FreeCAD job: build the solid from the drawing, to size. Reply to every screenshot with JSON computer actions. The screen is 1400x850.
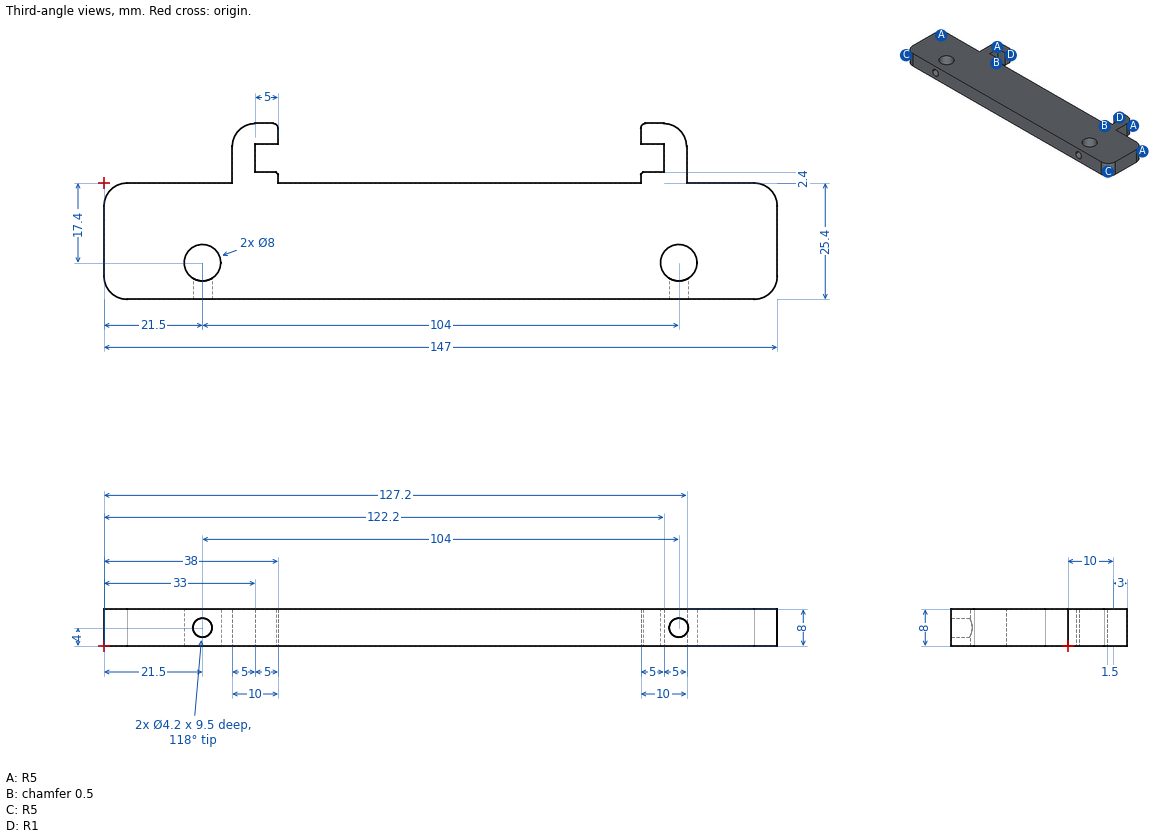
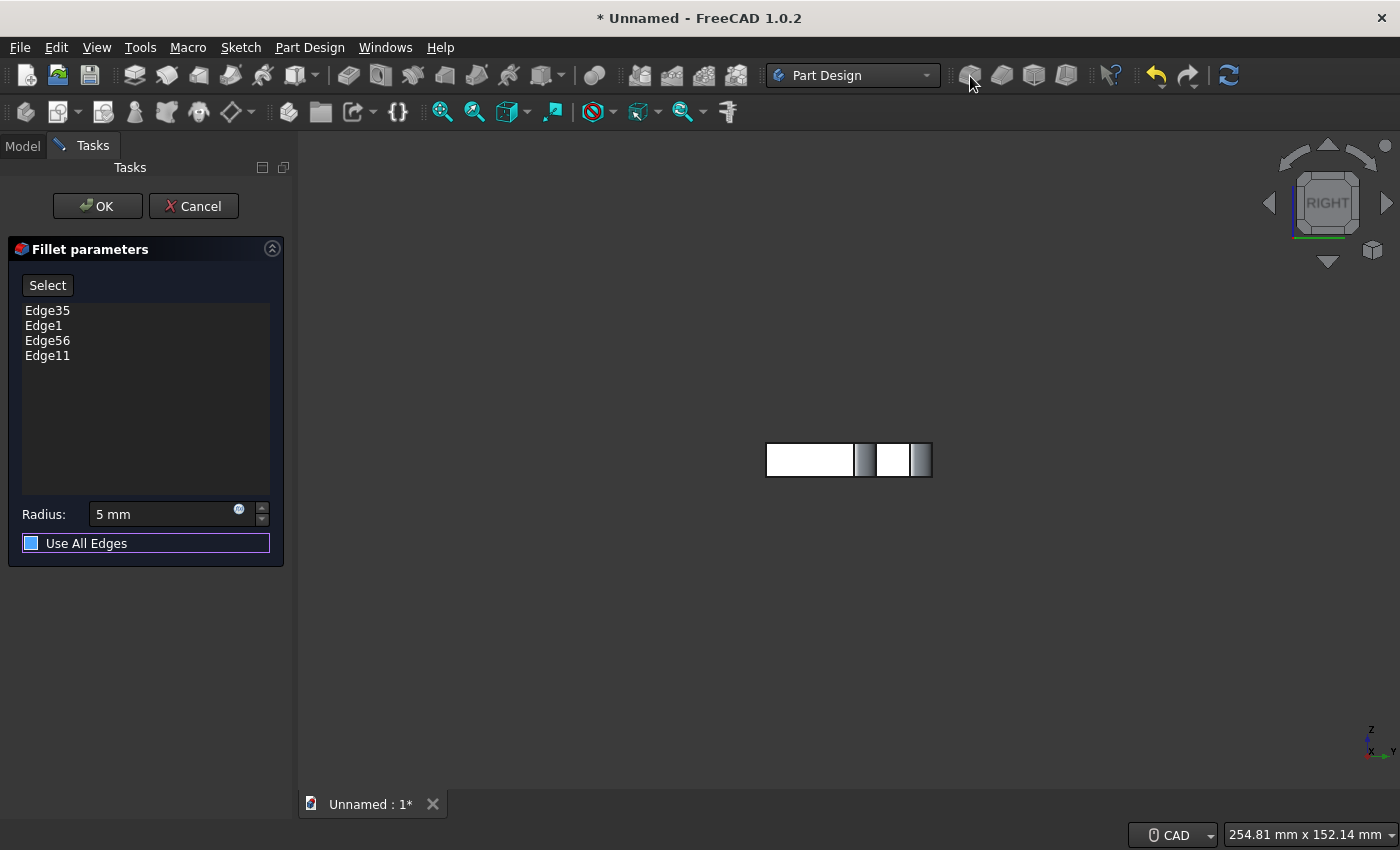
{"action": "left_click", "coordinate": [98, 206]}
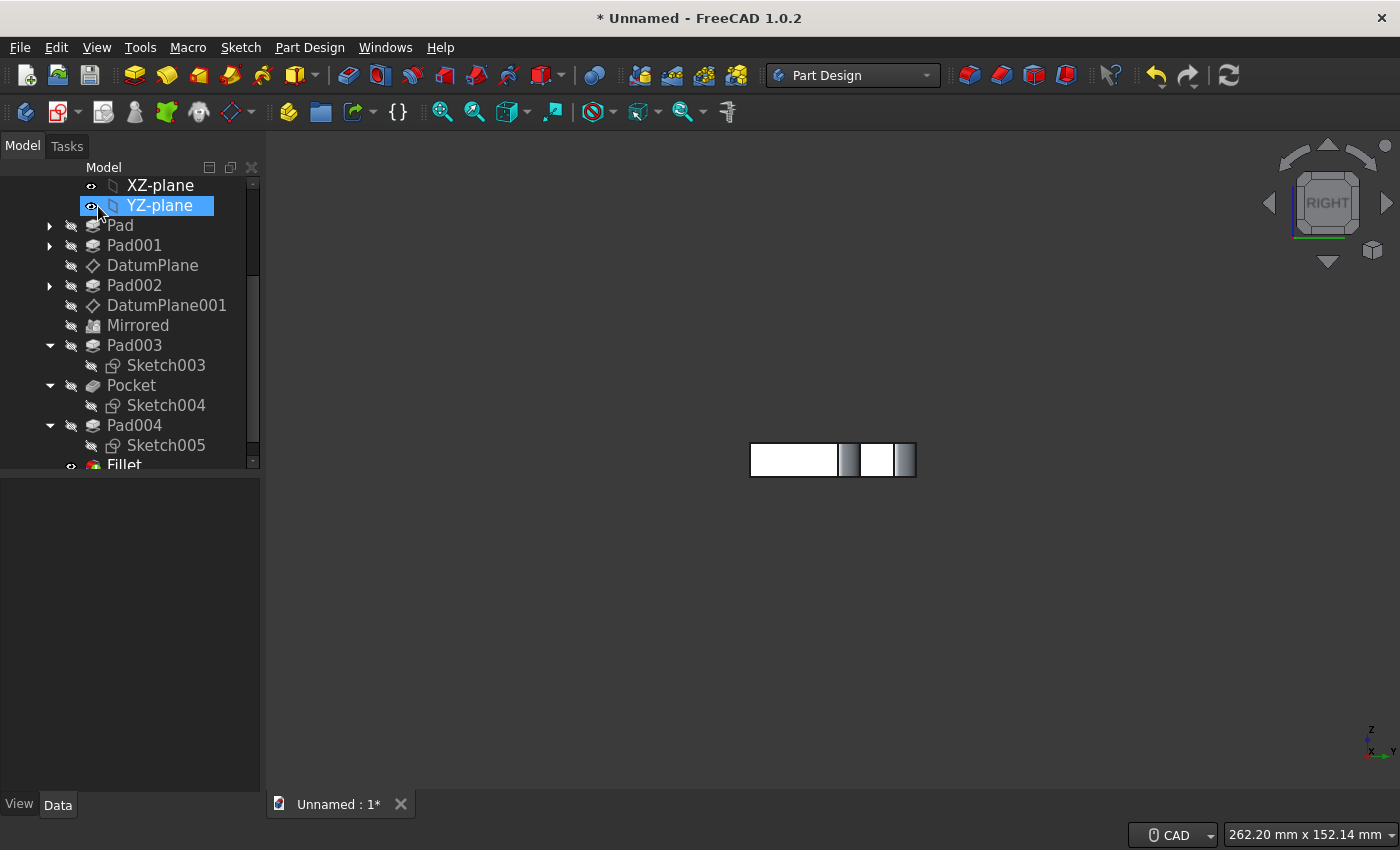
{"action": "left_click", "coordinate": [444, 112]}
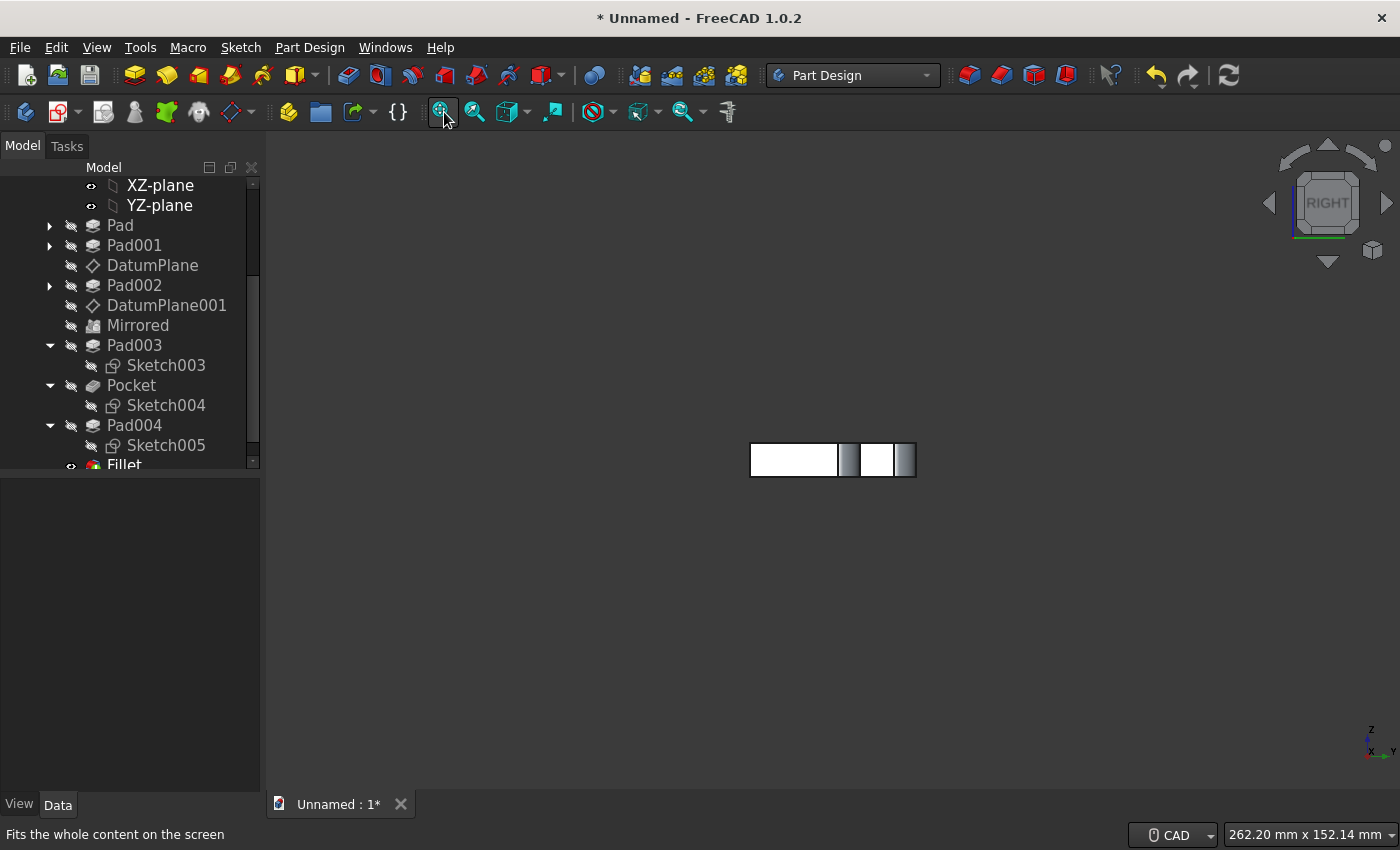
{"action": "key", "text": "0"}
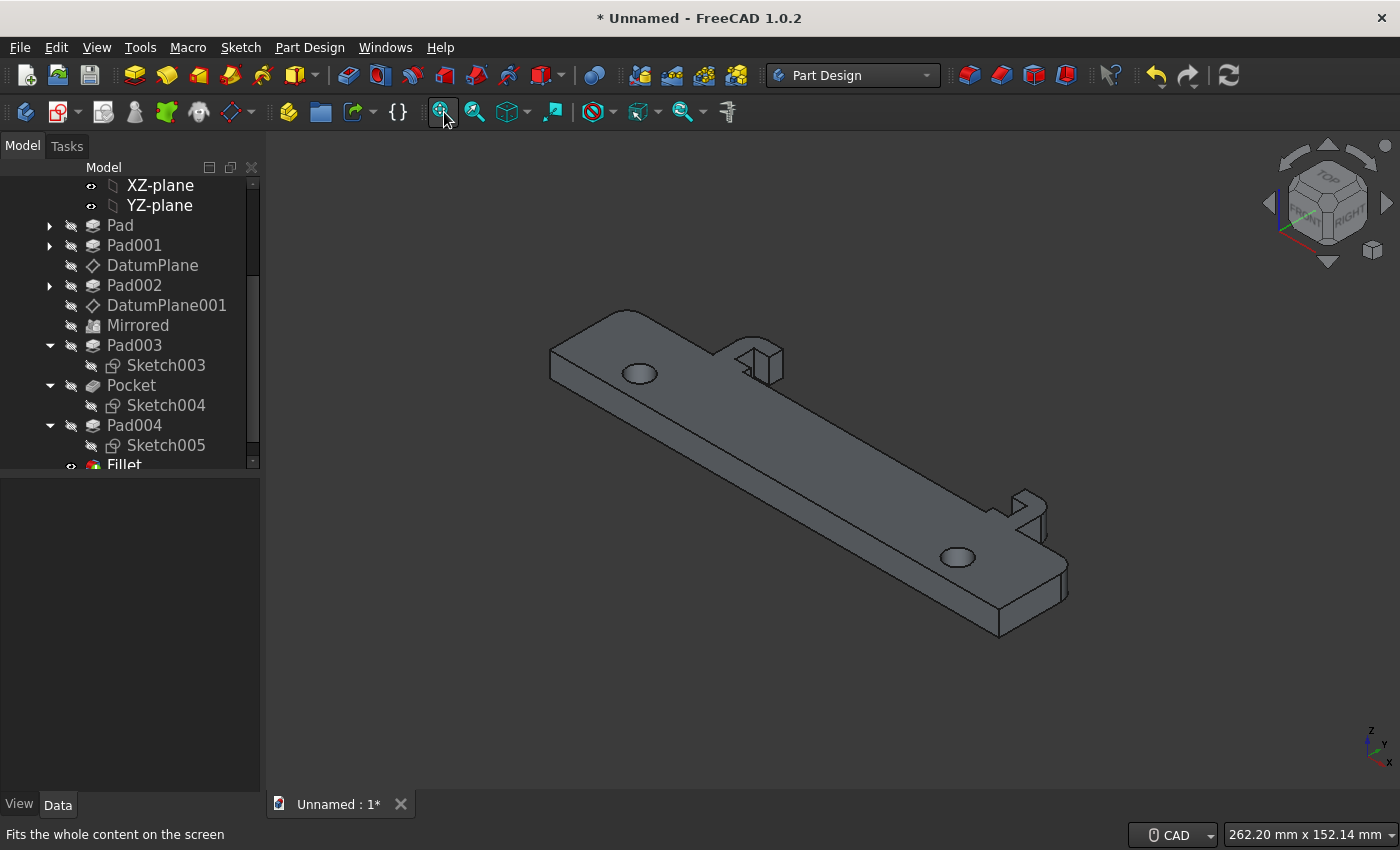
{"action": "key", "text": "2"}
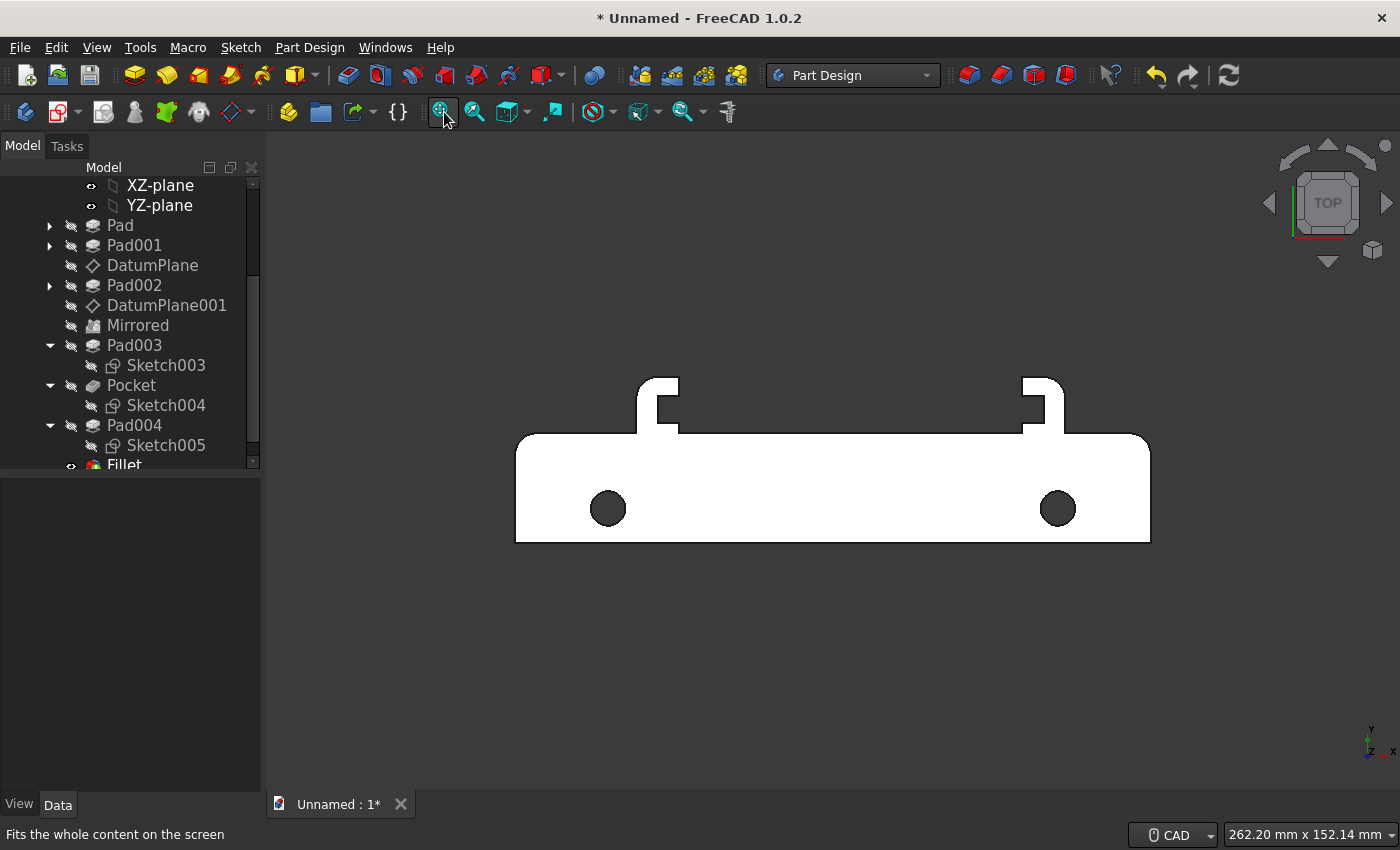
{"action": "key", "text": "1"}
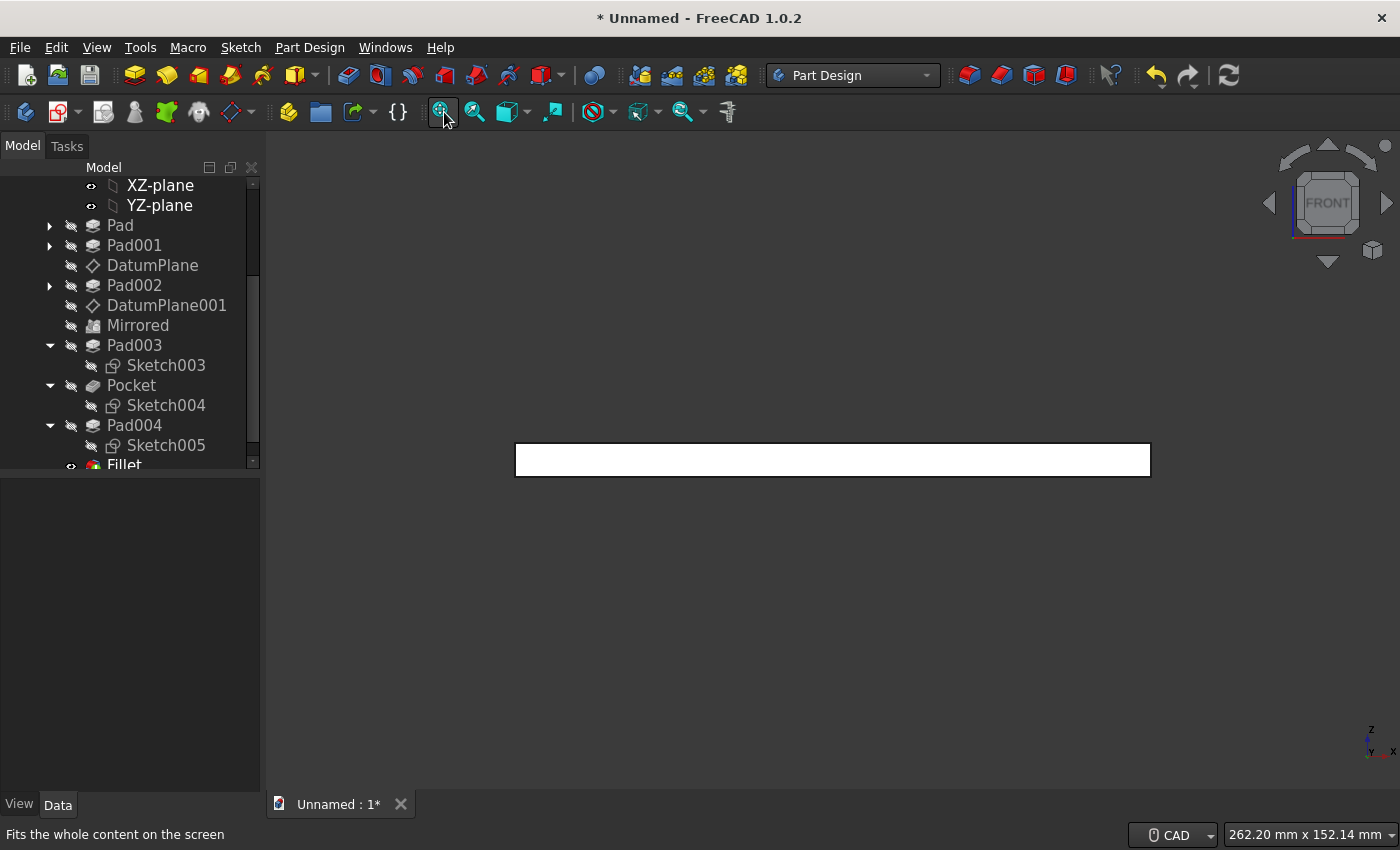
{"action": "key", "text": "3"}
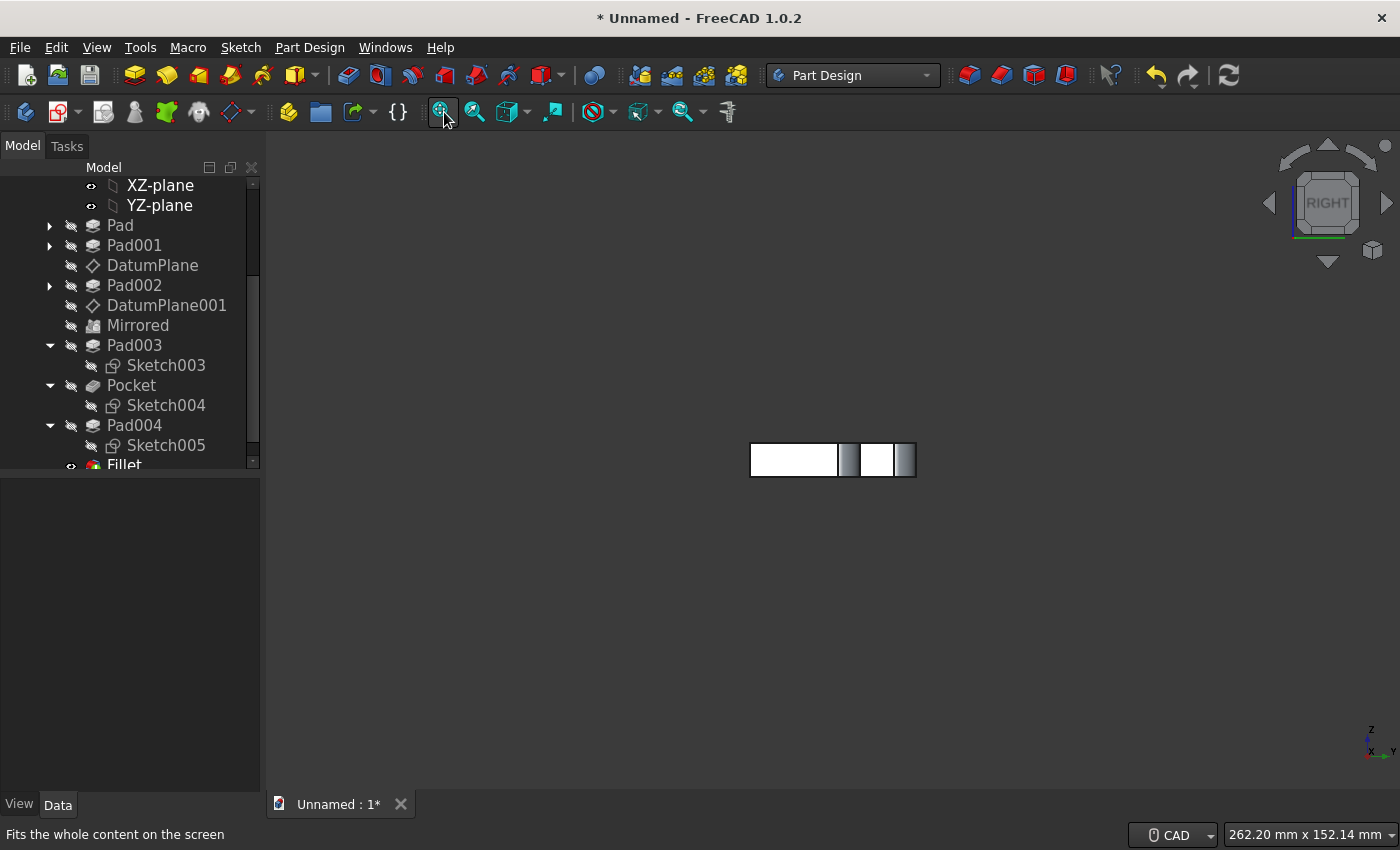
{"action": "left_click", "coordinate": [444, 112]}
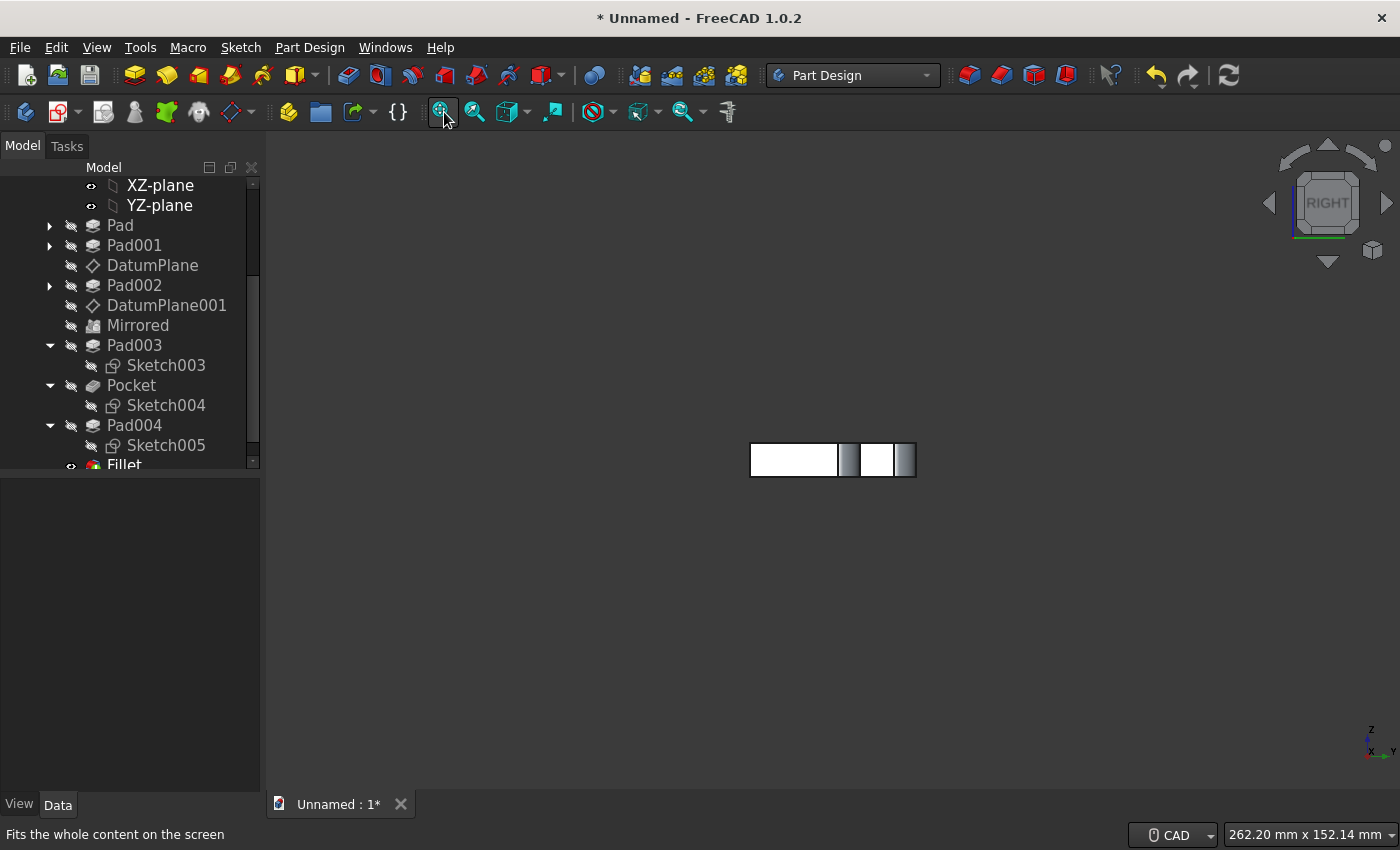
{"action": "key", "text": "5"}